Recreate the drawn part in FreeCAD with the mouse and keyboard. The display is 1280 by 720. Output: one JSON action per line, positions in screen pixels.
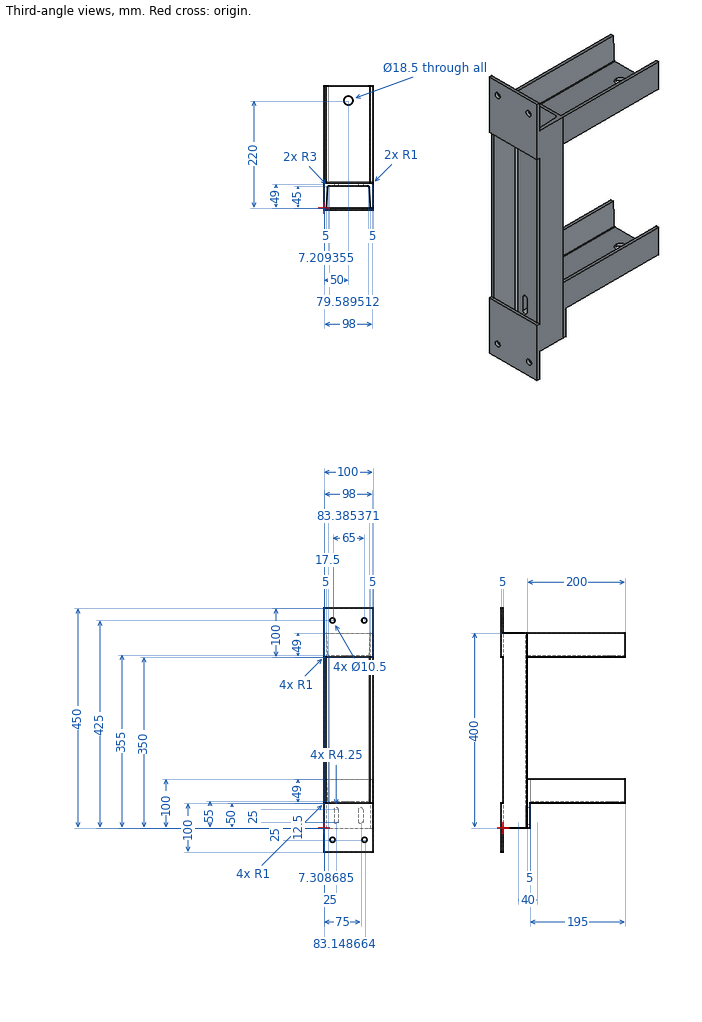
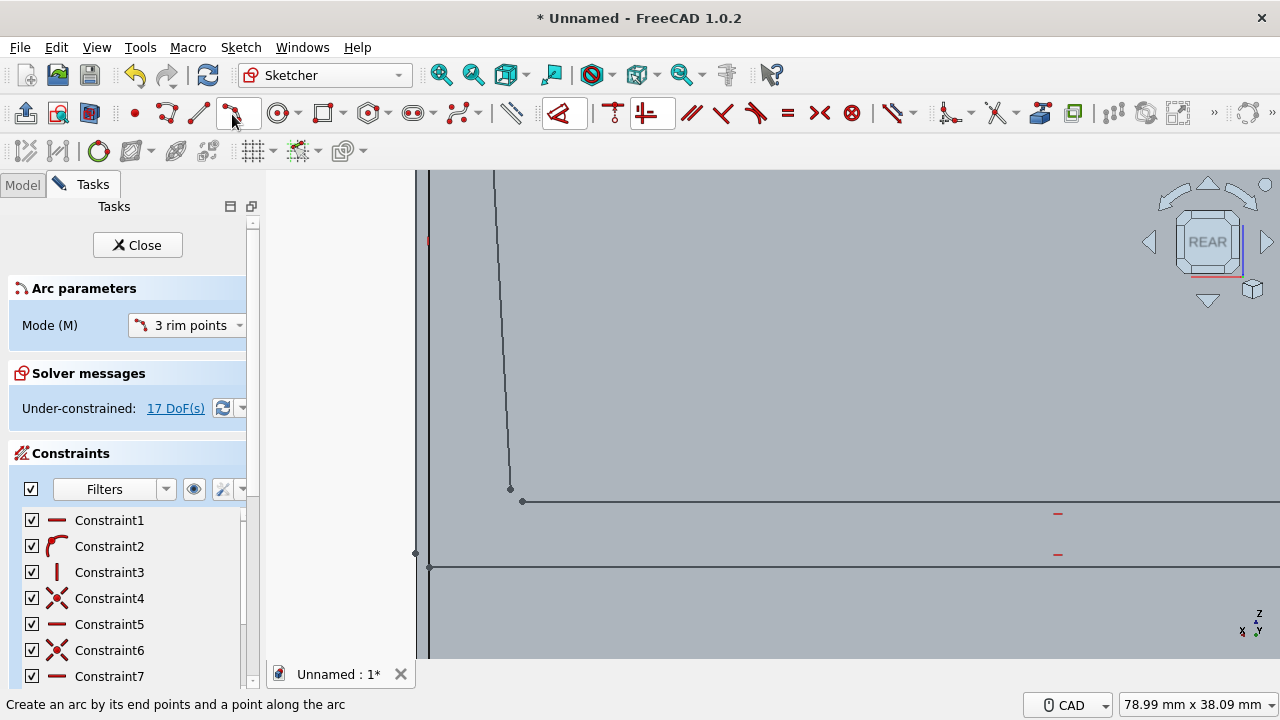
{"action": "scroll", "coordinate": [416, 553], "scroll_direction": "down", "scroll_amount": 4}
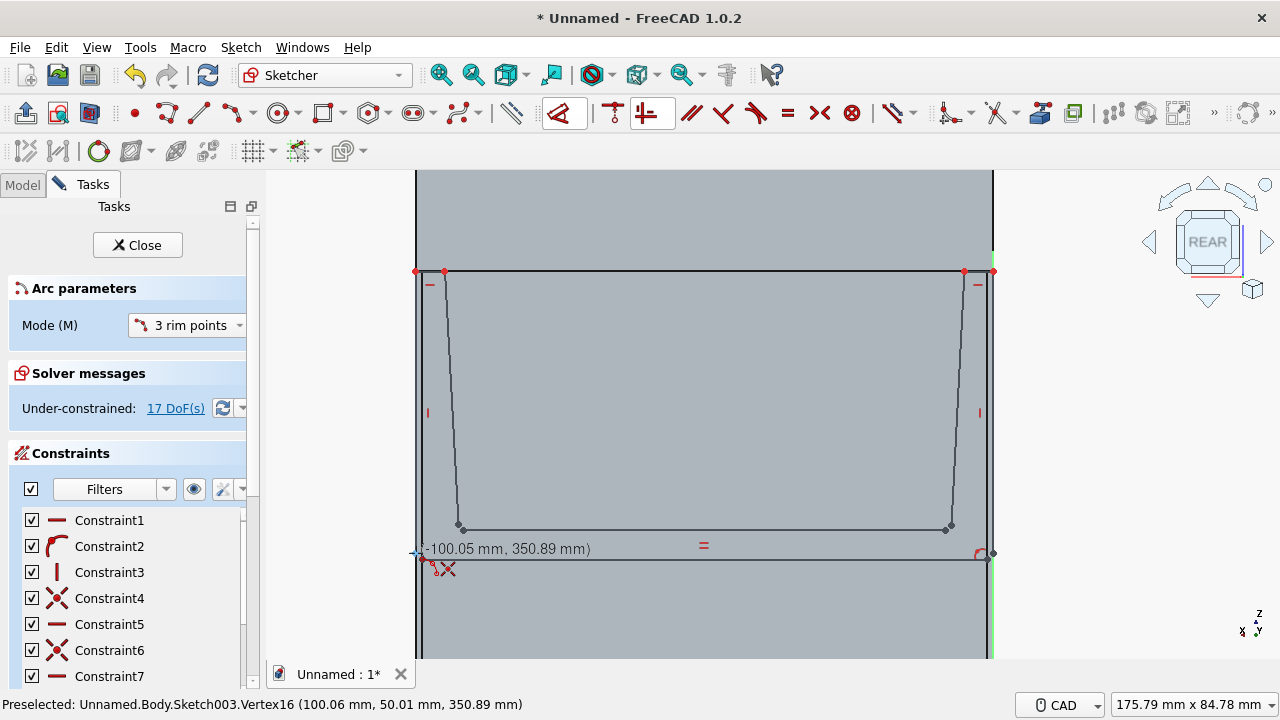
{"action": "scroll", "coordinate": [987, 559], "scroll_direction": "up", "scroll_amount": 6}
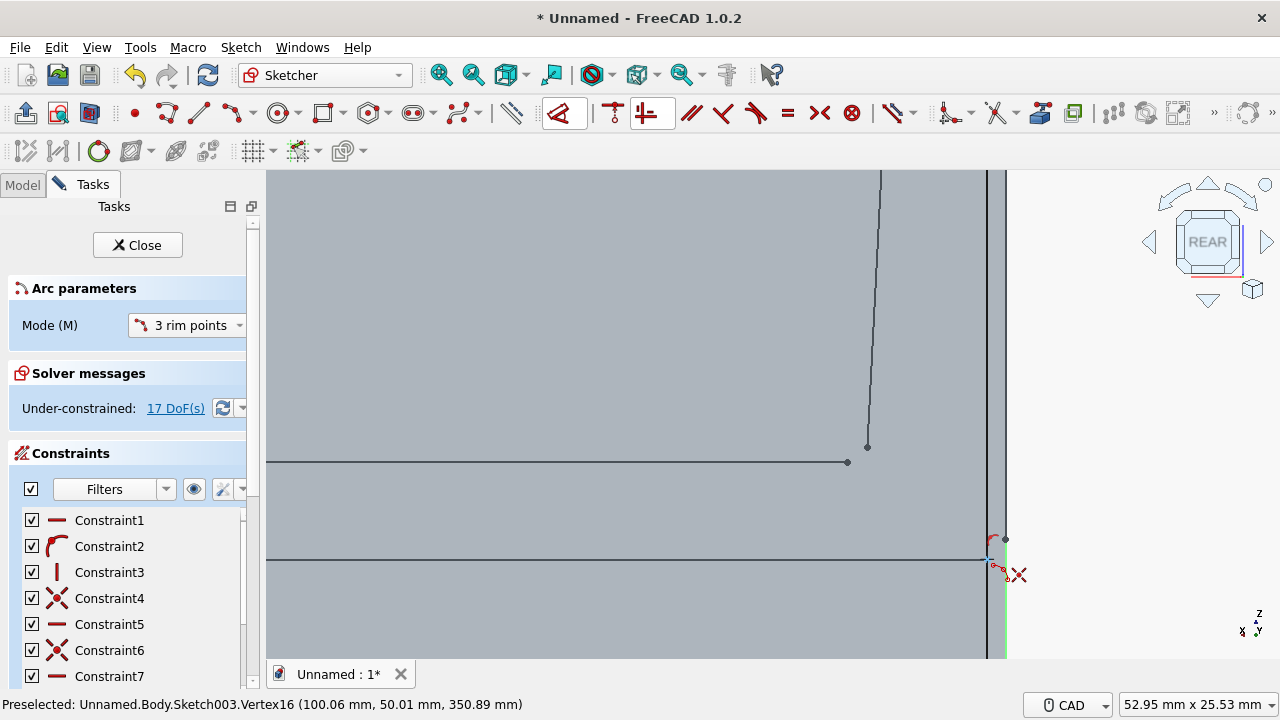
{"action": "left_click", "coordinate": [987, 560]}
{"action": "left_click", "coordinate": [1006, 539]}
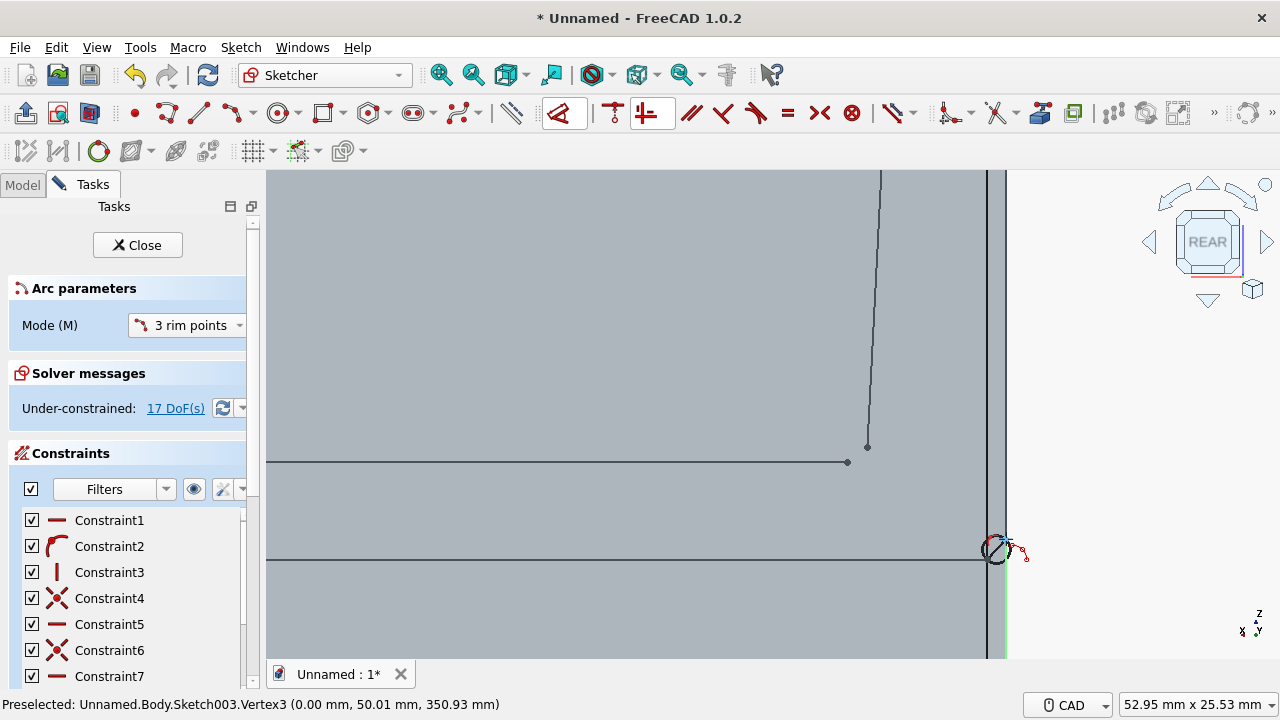
{"action": "scroll", "coordinate": [1000, 552], "scroll_direction": "up", "scroll_amount": 6}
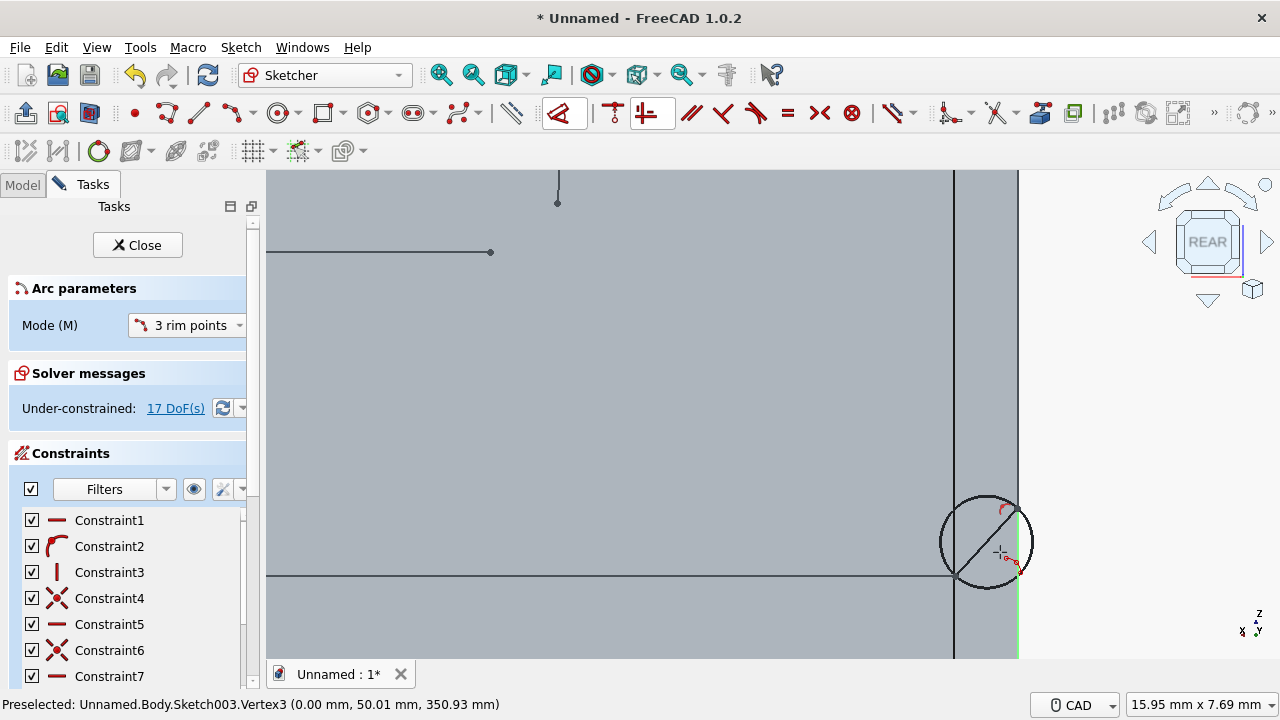
{"action": "left_click", "coordinate": [999, 549]}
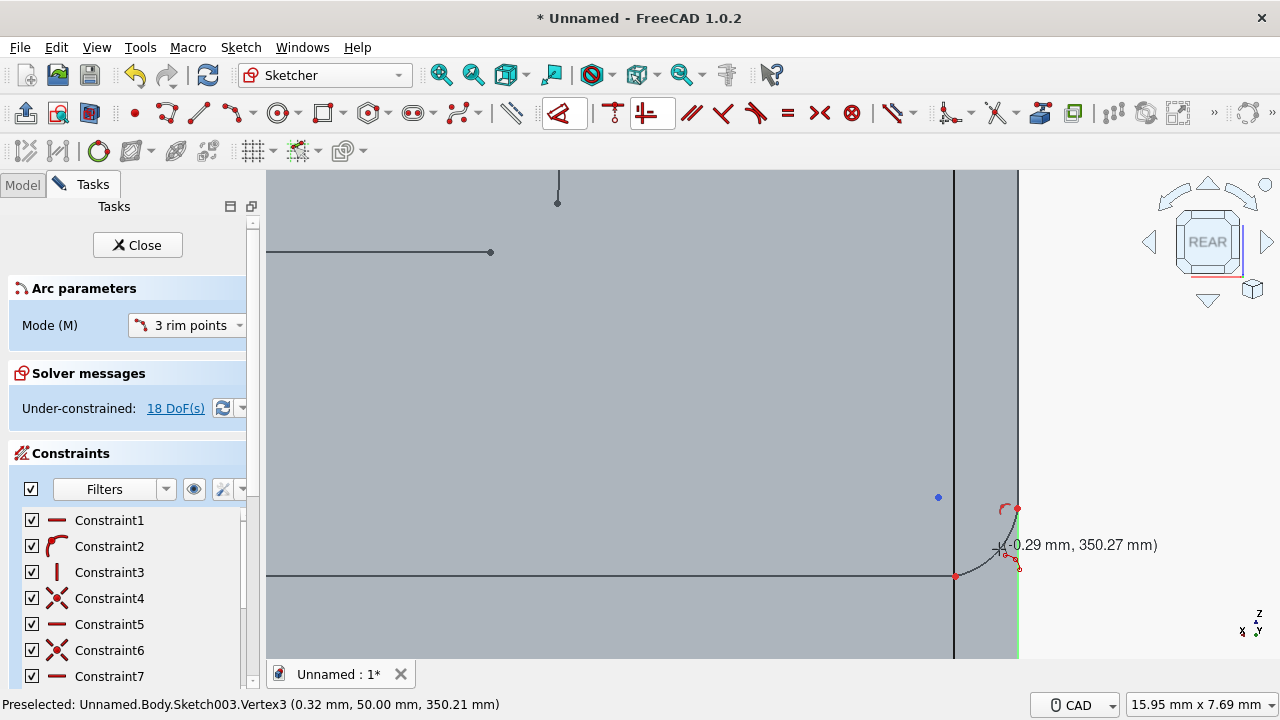
{"action": "scroll", "coordinate": [990, 558], "scroll_direction": "down", "scroll_amount": 12}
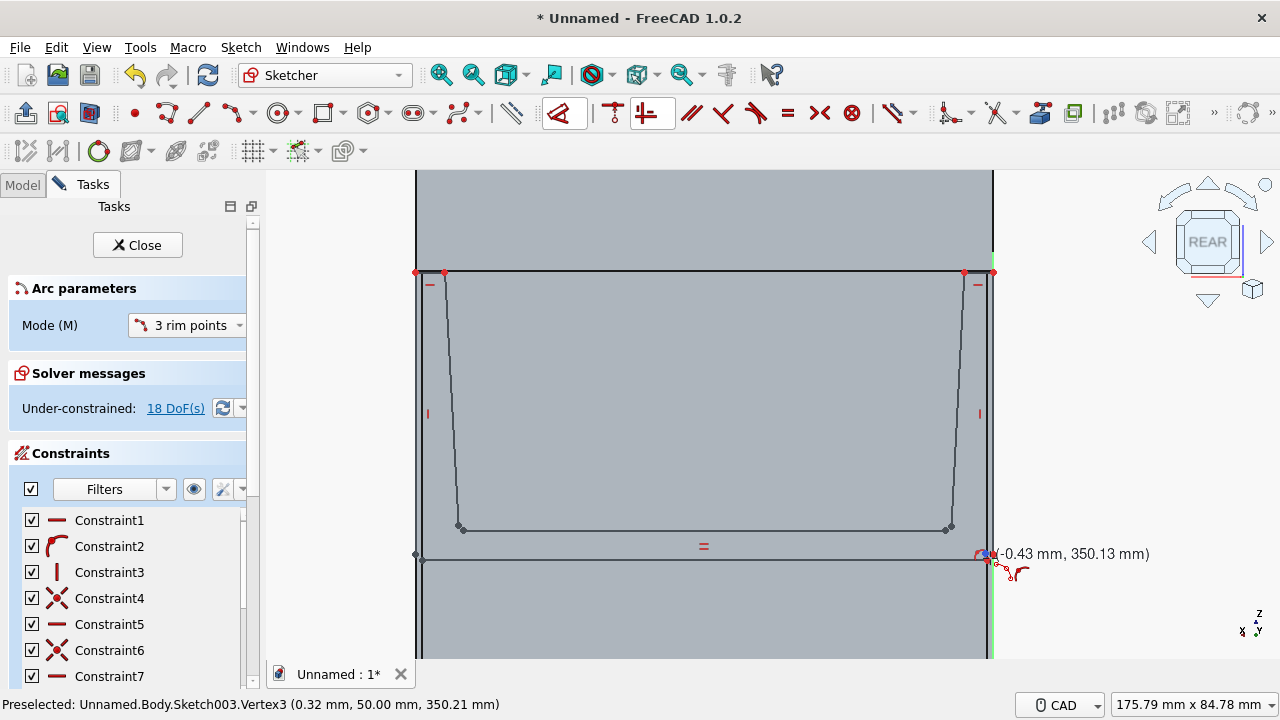
{"action": "scroll", "coordinate": [951, 525], "scroll_direction": "up", "scroll_amount": 4}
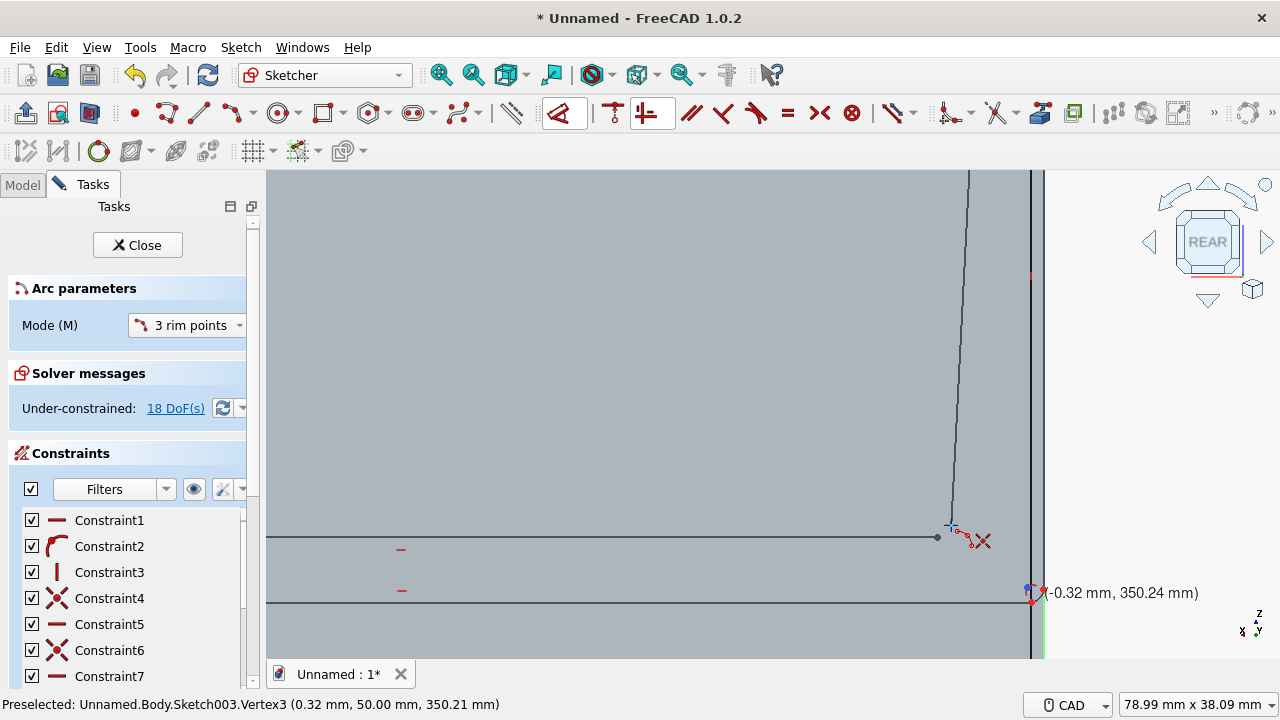
{"action": "left_click", "coordinate": [951, 528]}
{"action": "left_click", "coordinate": [938, 537]}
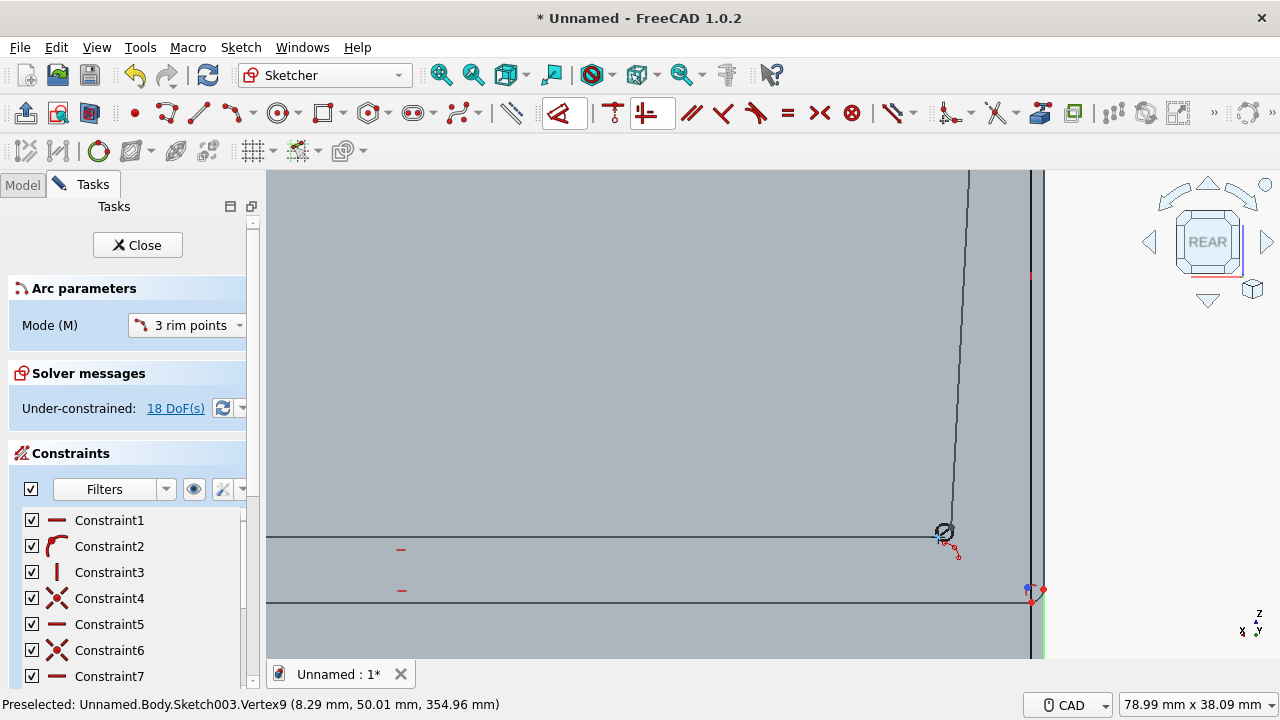
{"action": "scroll", "coordinate": [946, 533], "scroll_direction": "up", "scroll_amount": 8}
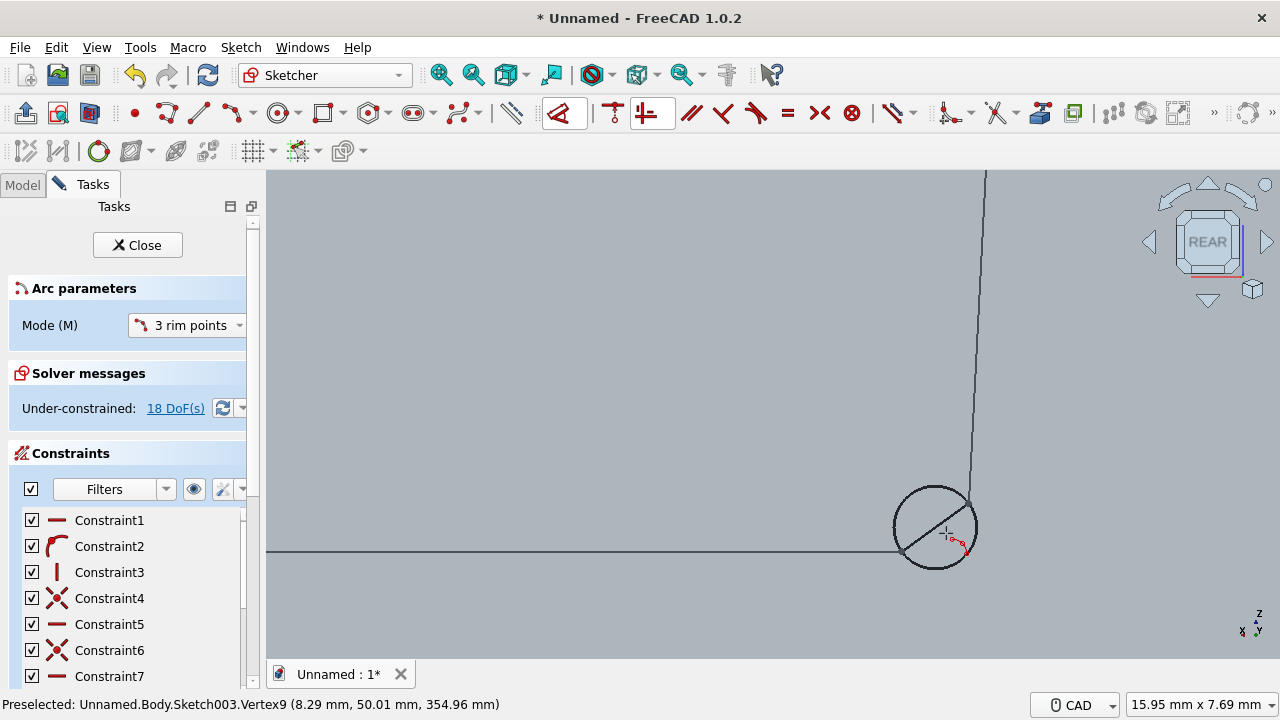
{"action": "left_click", "coordinate": [944, 532]}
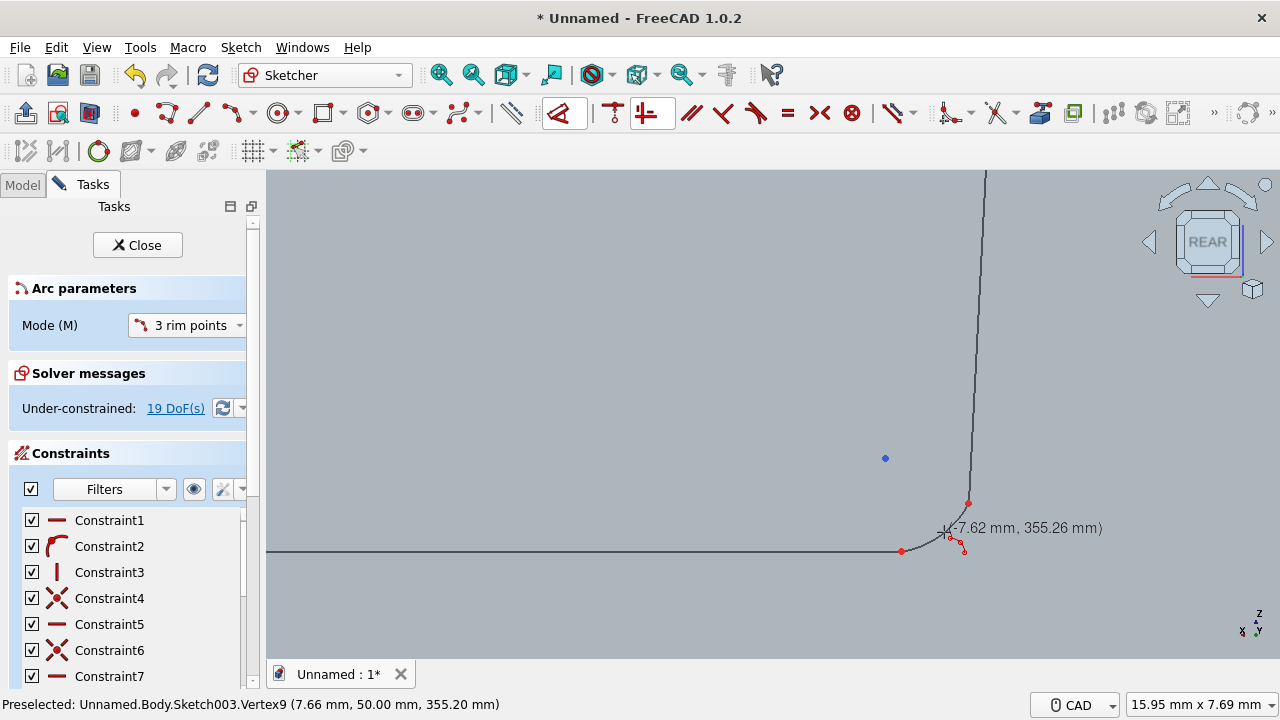
{"action": "scroll", "coordinate": [949, 528], "scroll_direction": "down", "scroll_amount": 12}